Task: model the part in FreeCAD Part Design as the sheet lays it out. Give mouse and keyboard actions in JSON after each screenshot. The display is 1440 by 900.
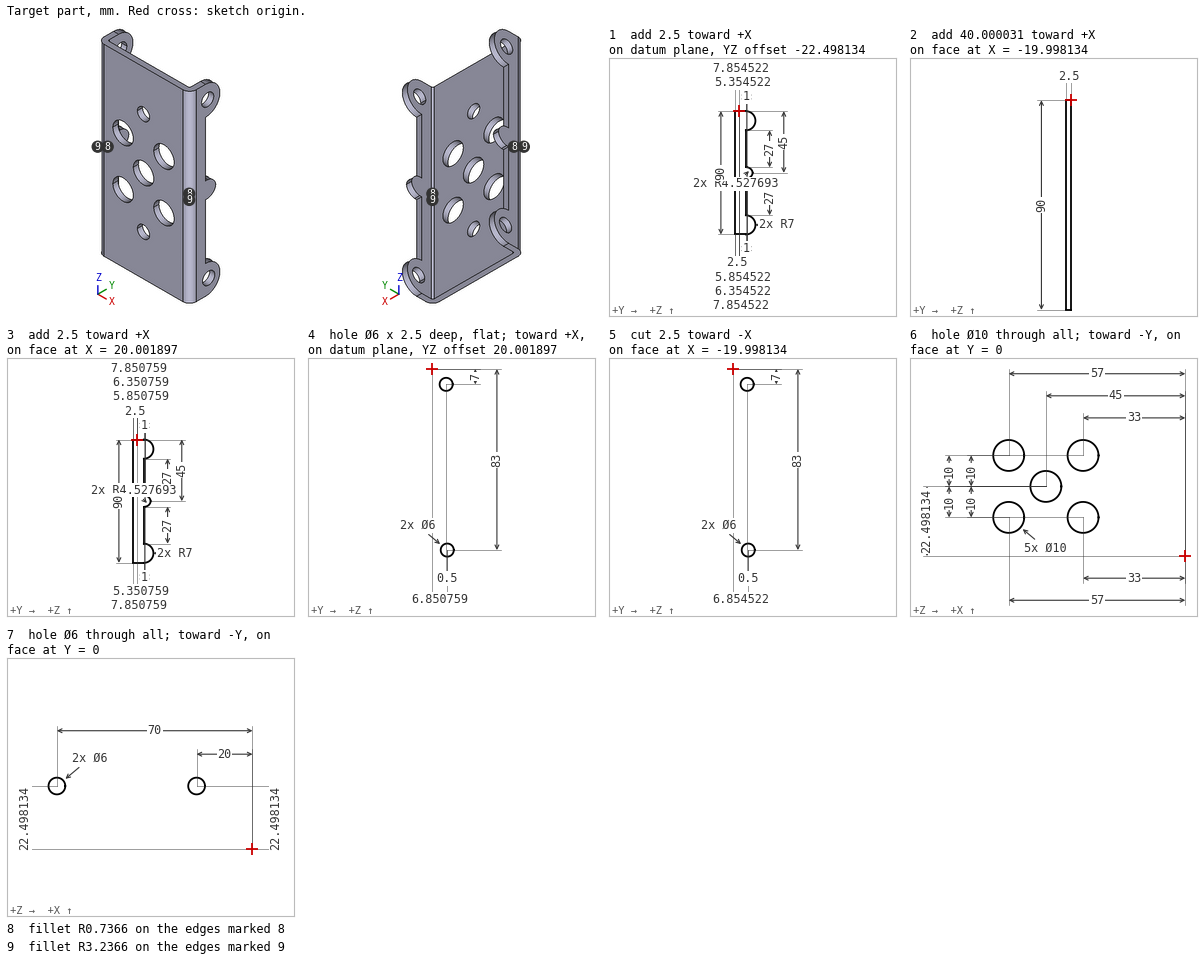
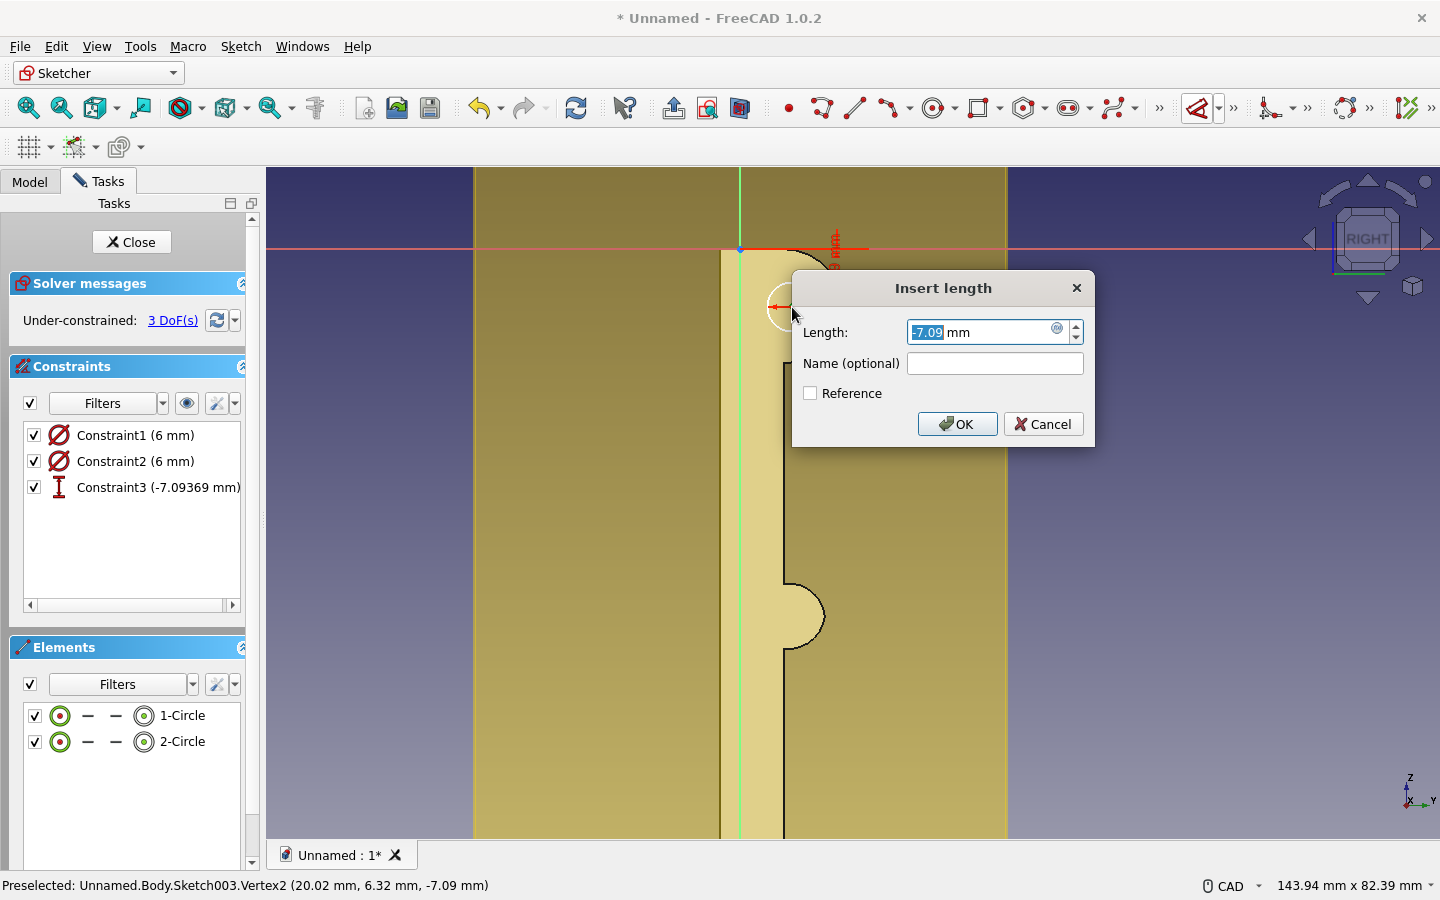
{"action": "type", "text": "-7"}
{"action": "key", "text": "Return"}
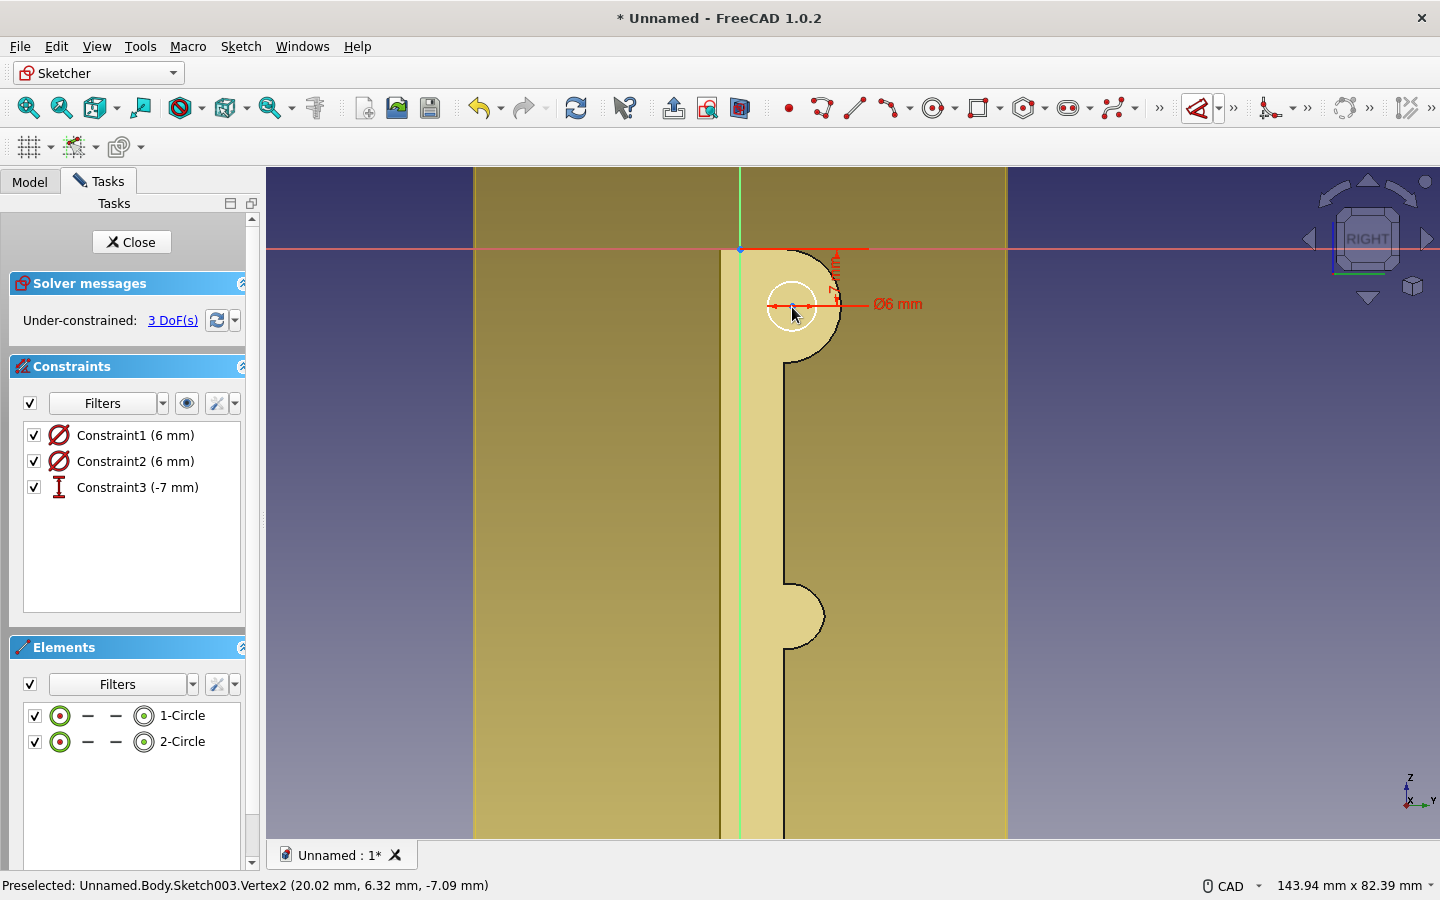
{"action": "scroll", "coordinate": [792, 306], "scroll_direction": "down", "scroll_amount": 2}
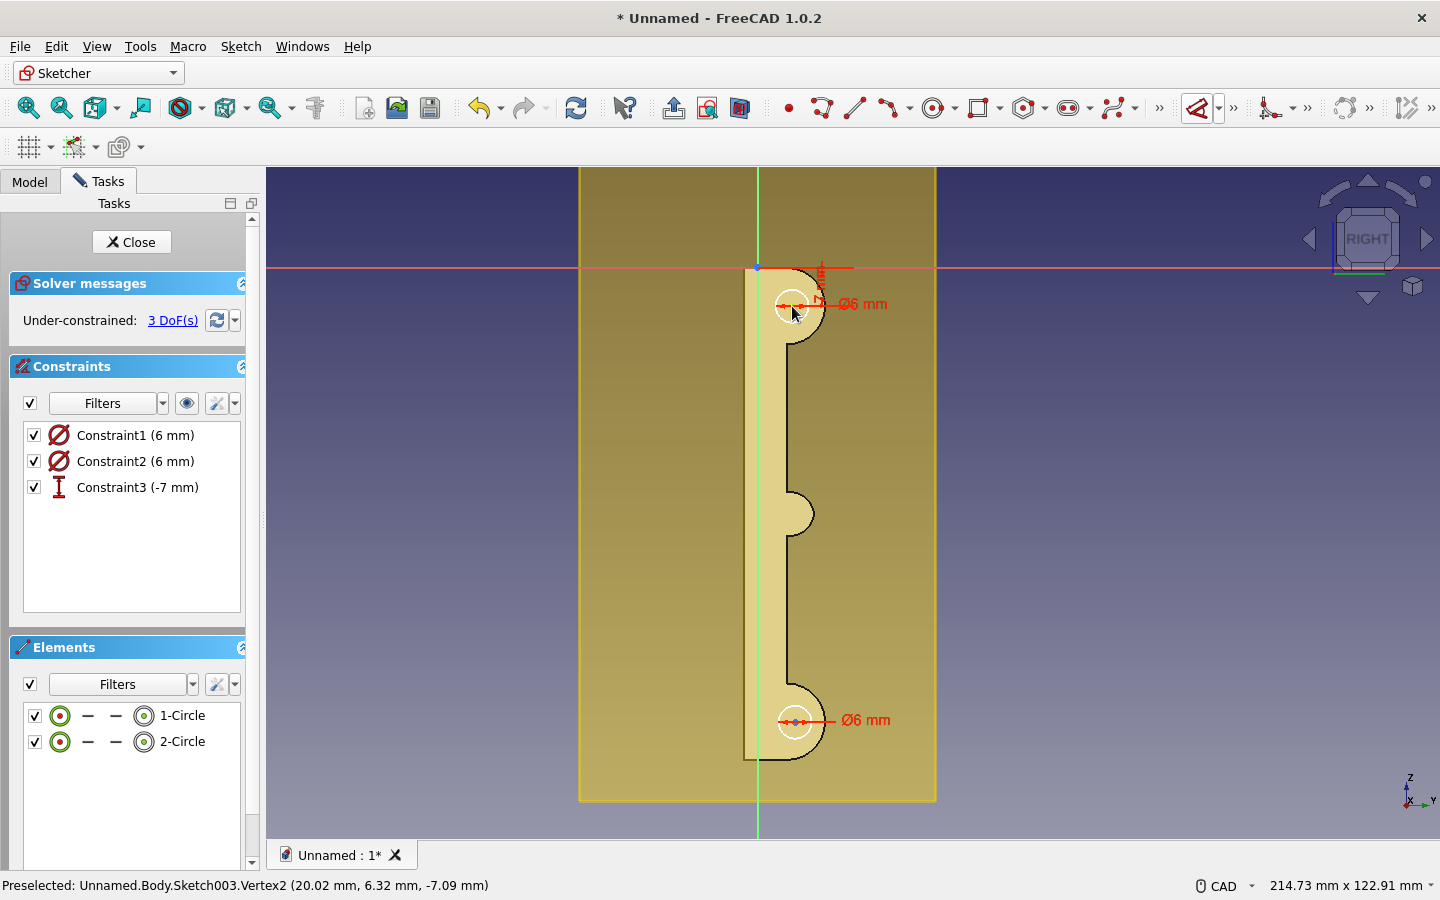
{"action": "left_click", "coordinate": [795, 722]}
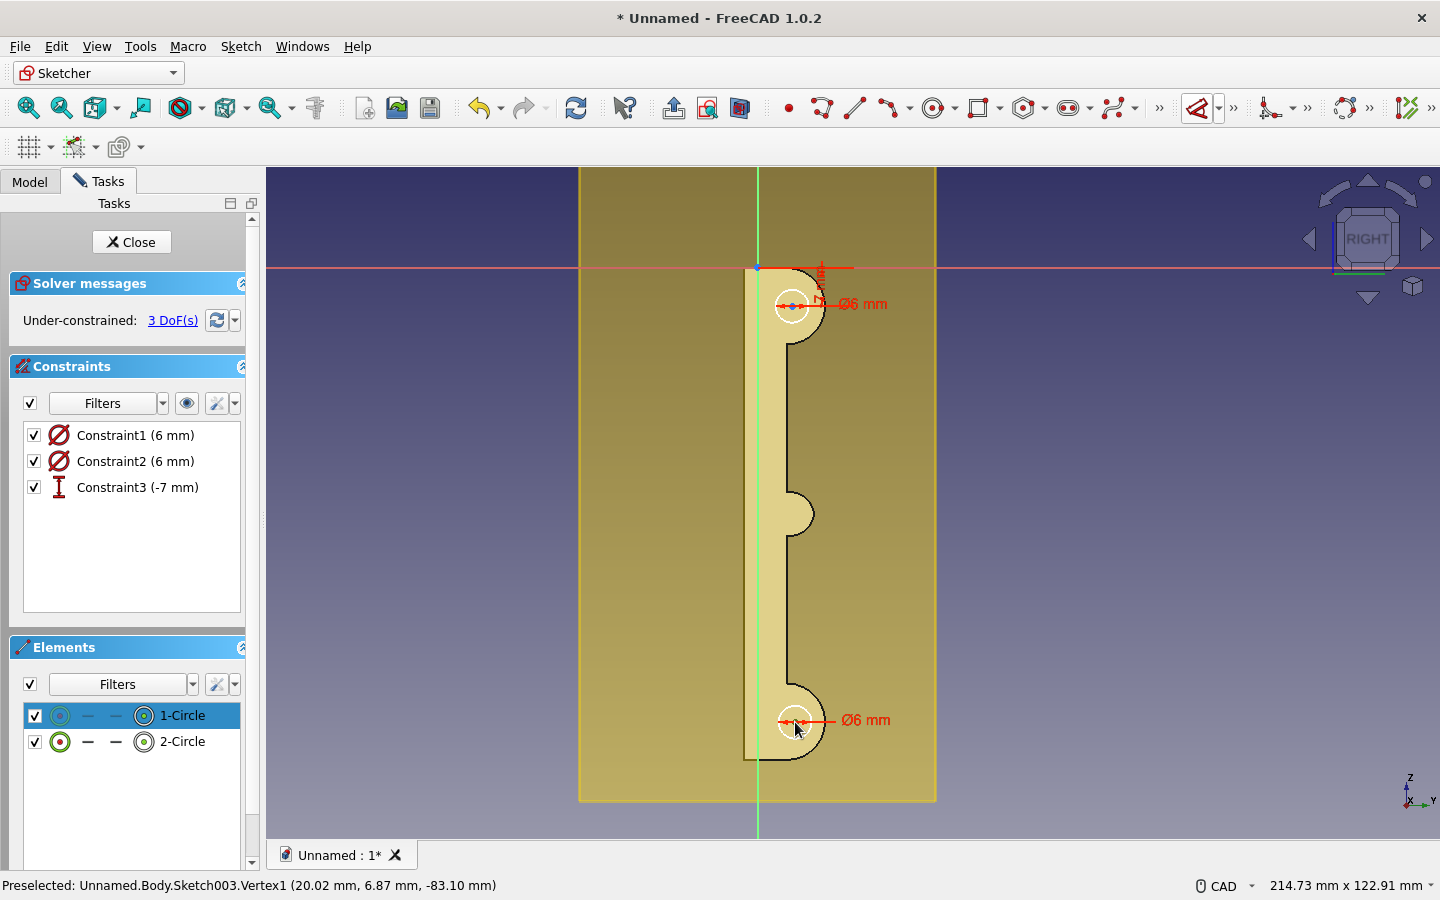
{"action": "left_click", "coordinate": [1218, 108]}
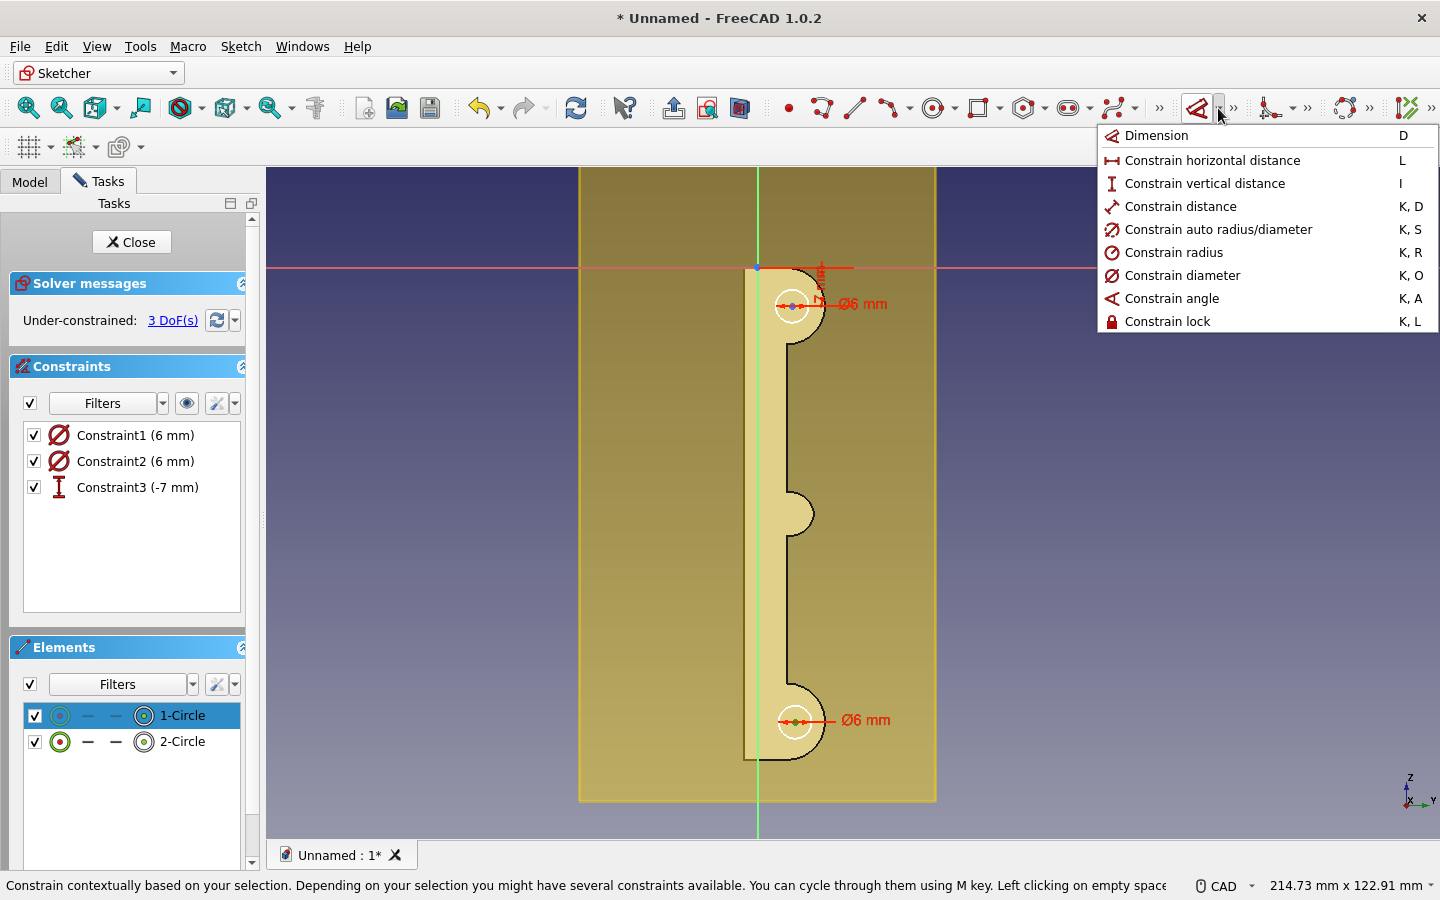
{"action": "left_click", "coordinate": [1268, 184]}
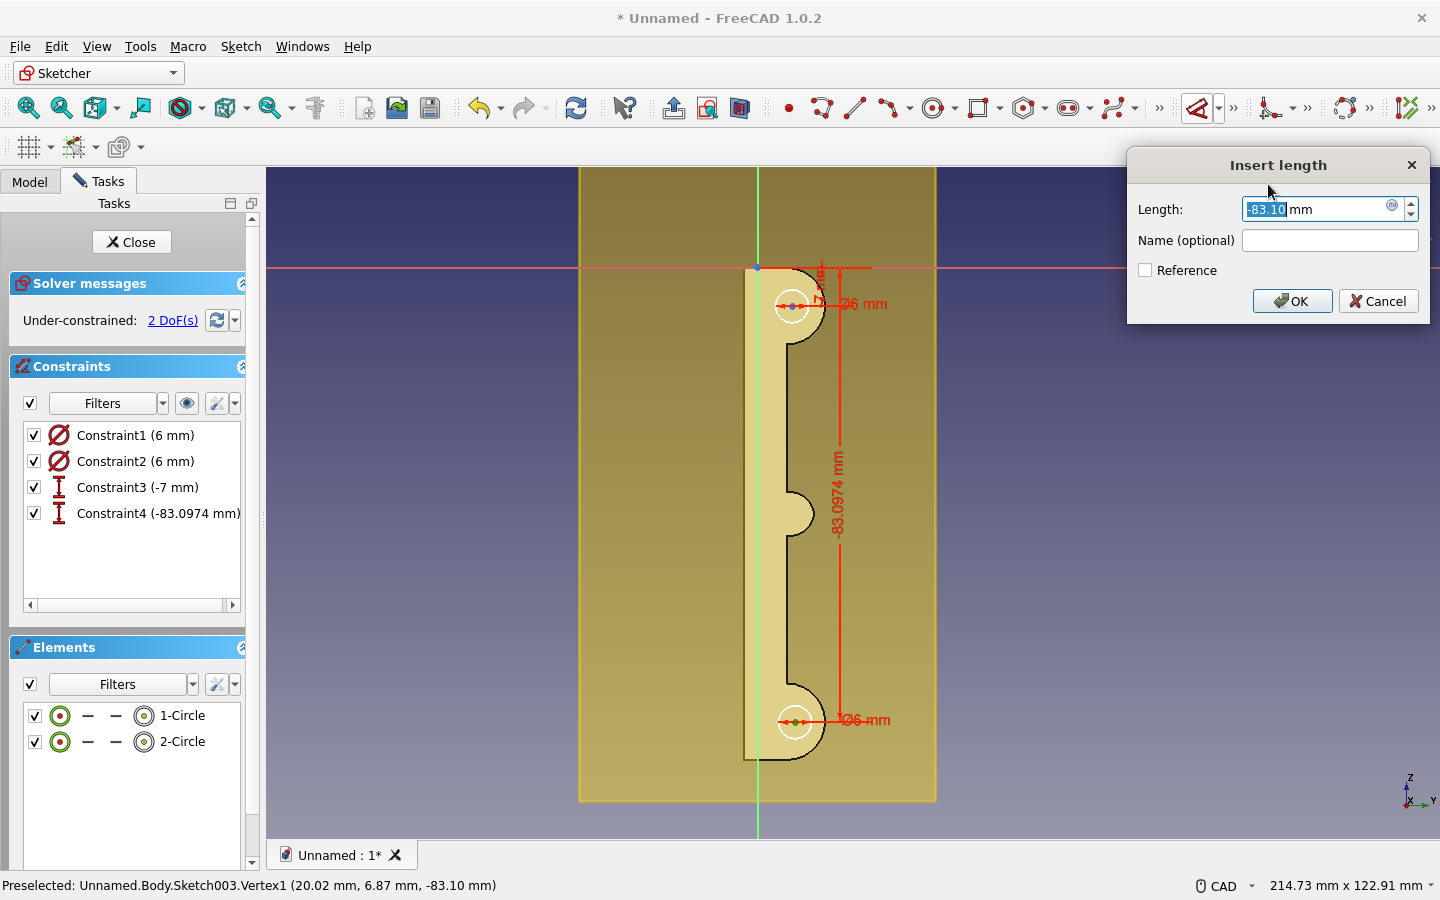
{"action": "type", "text": "-83"}
{"action": "key", "text": "Return"}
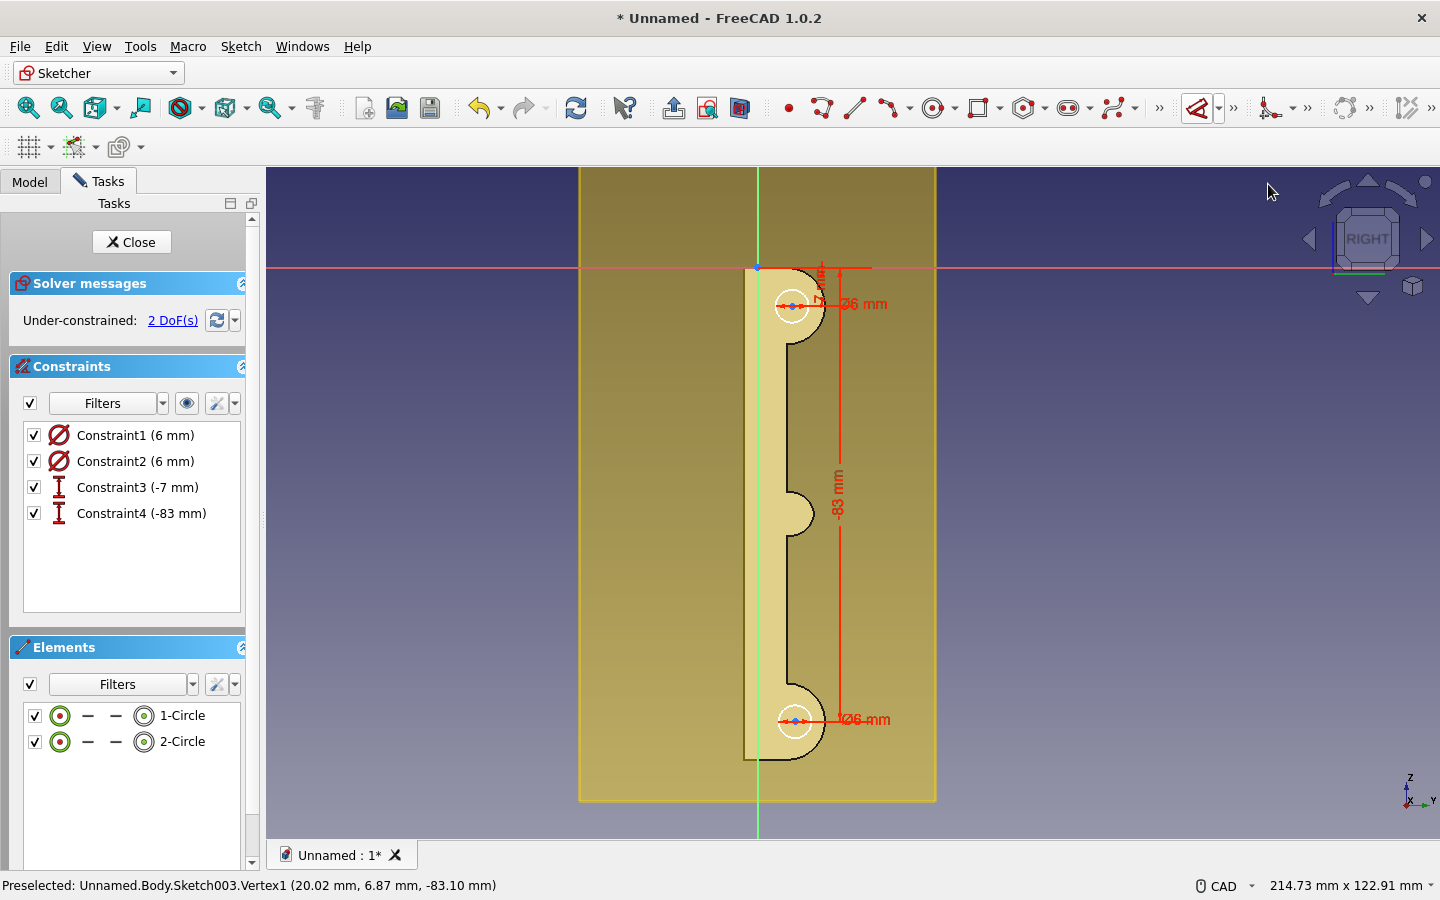
{"action": "scroll", "coordinate": [795, 722], "scroll_direction": "up", "scroll_amount": 14}